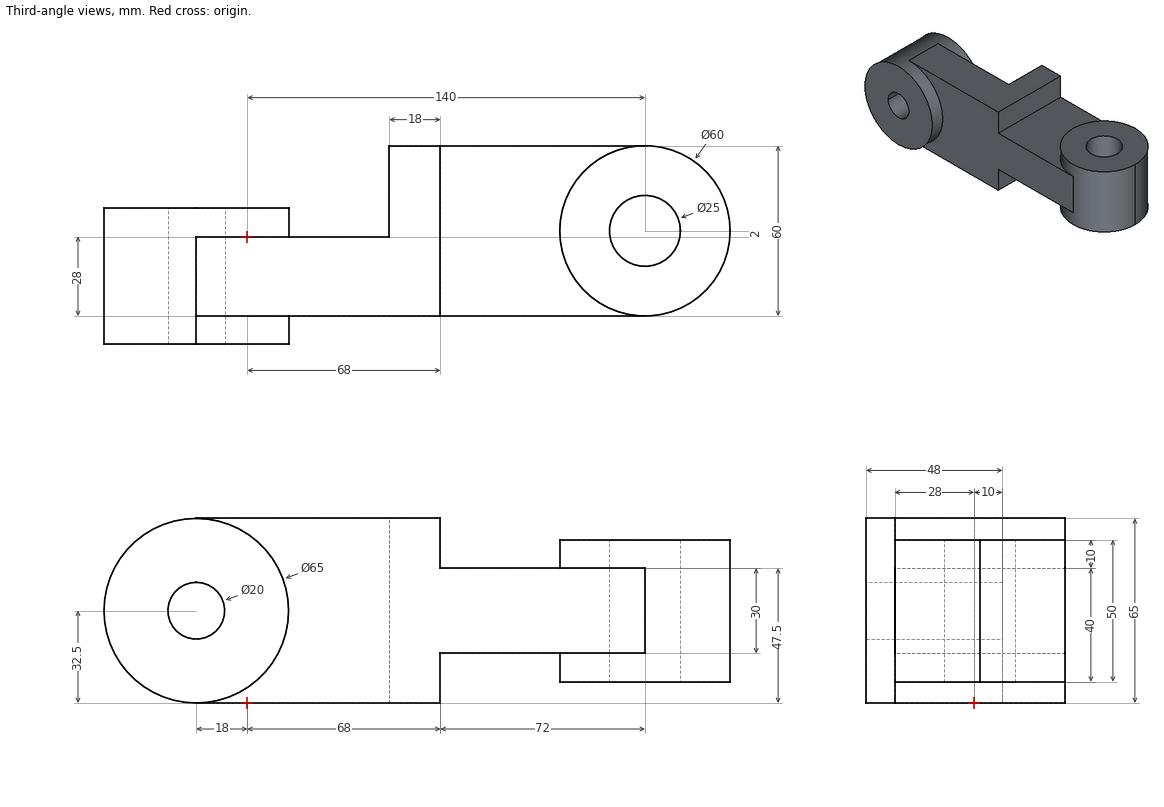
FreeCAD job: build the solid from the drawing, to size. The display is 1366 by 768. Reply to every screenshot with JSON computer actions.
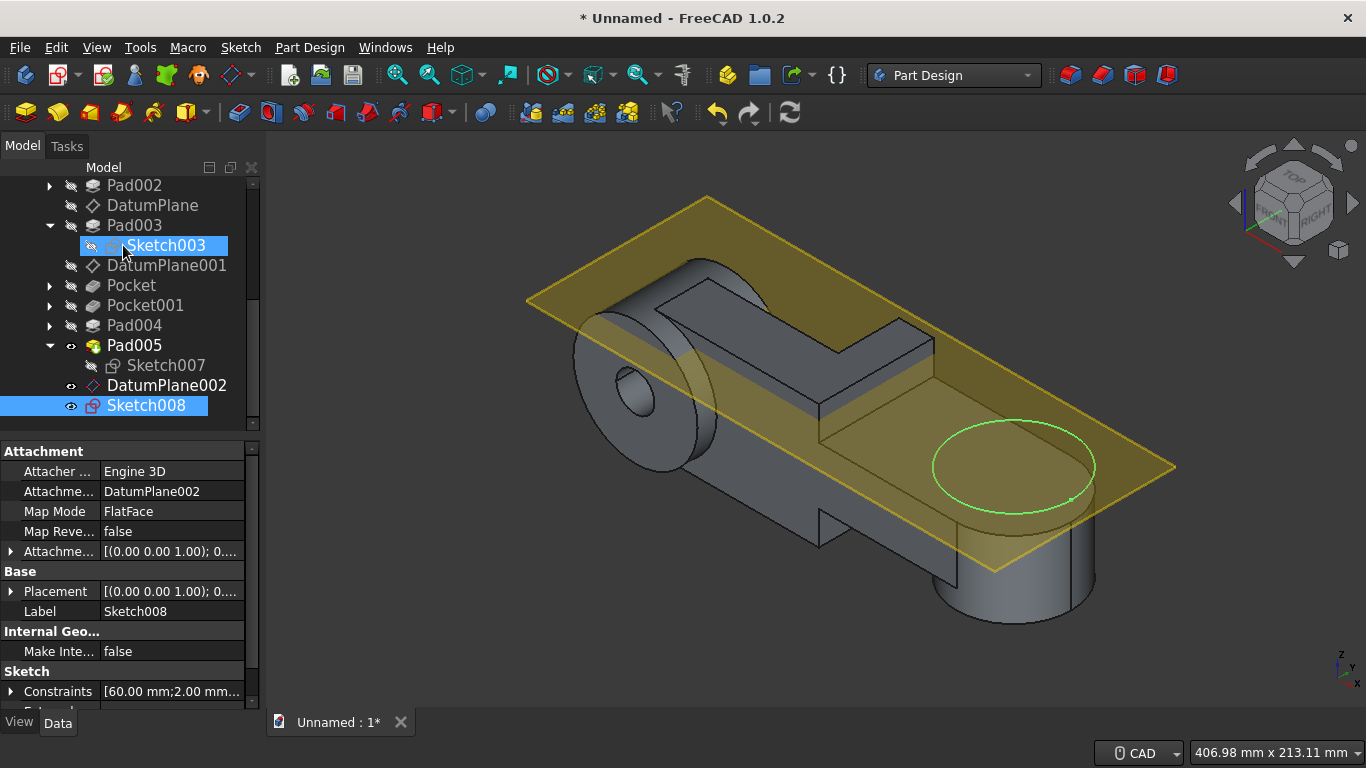
{"action": "left_click", "coordinate": [26, 112]}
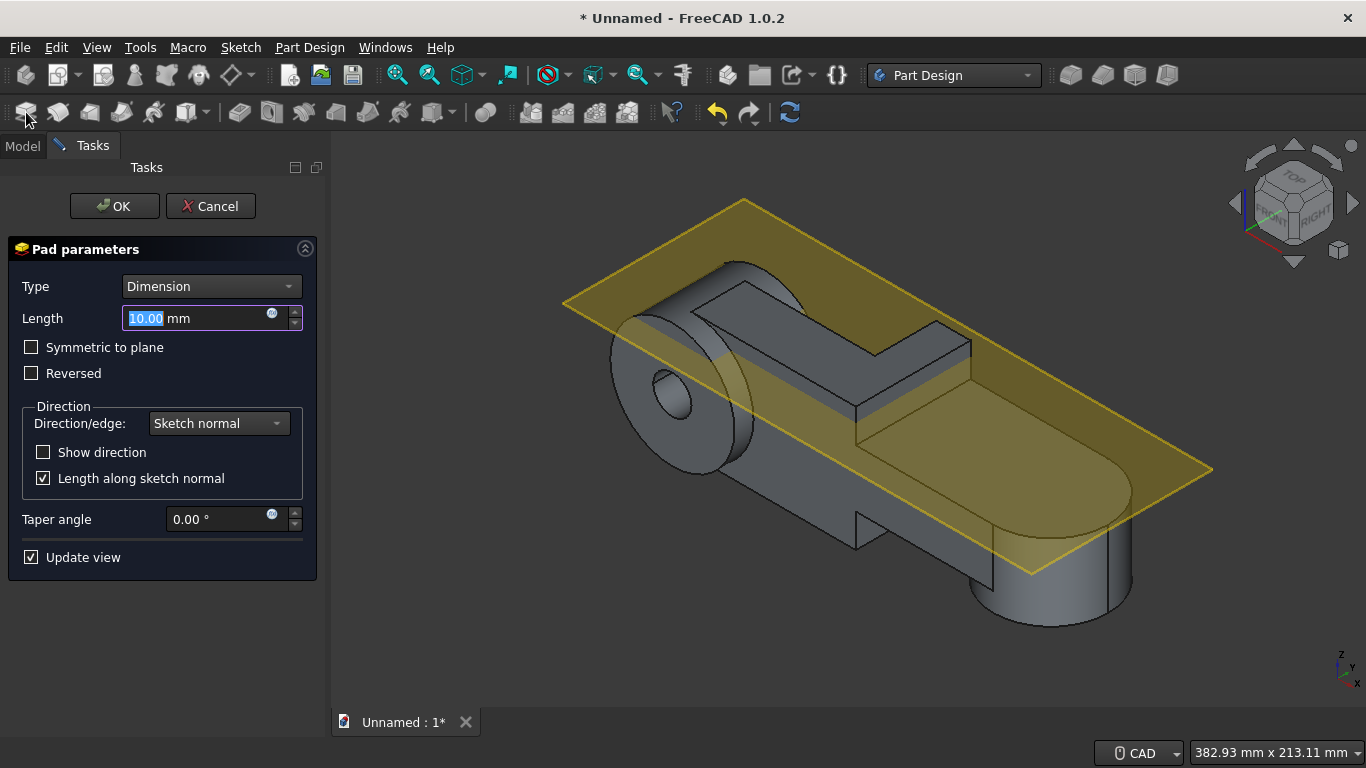
{"action": "type", "text": "10"}
{"action": "key", "text": "Tab"}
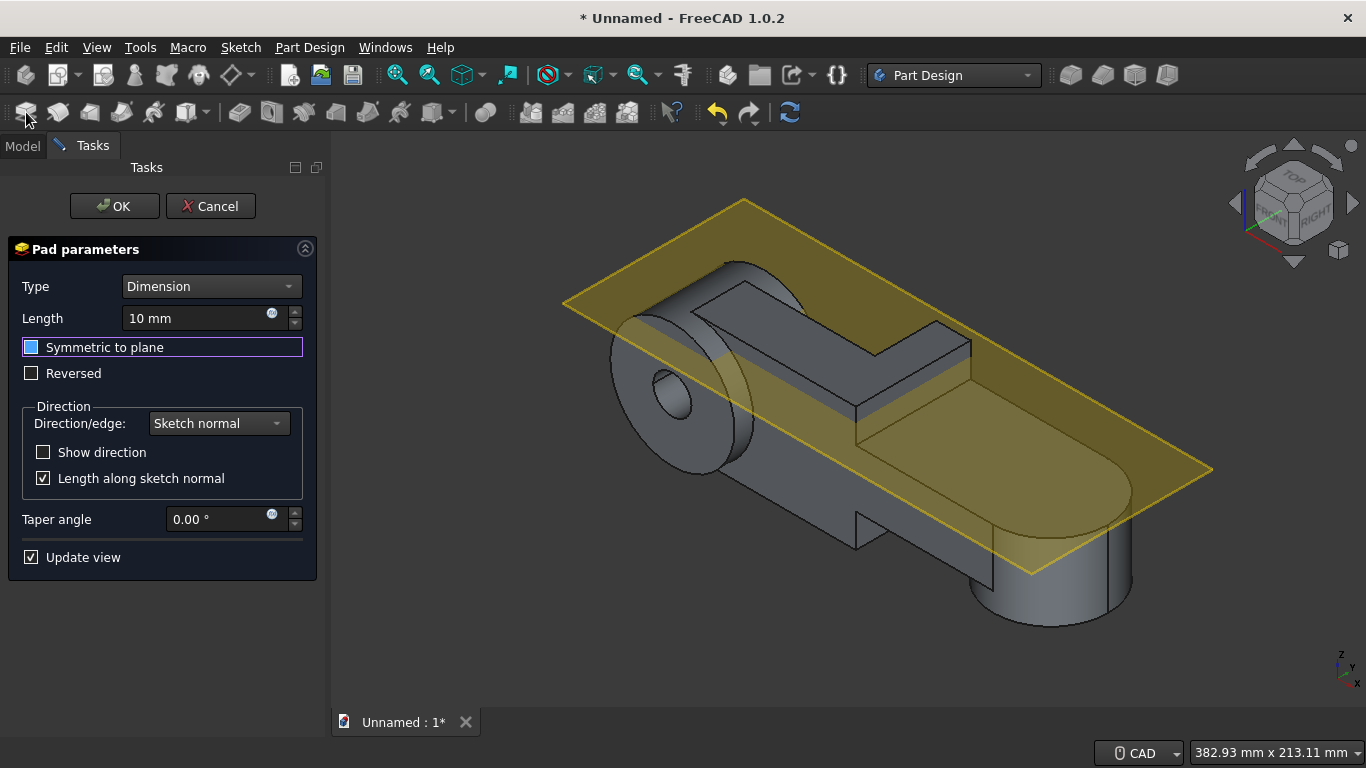
{"action": "left_click", "coordinate": [30, 373]}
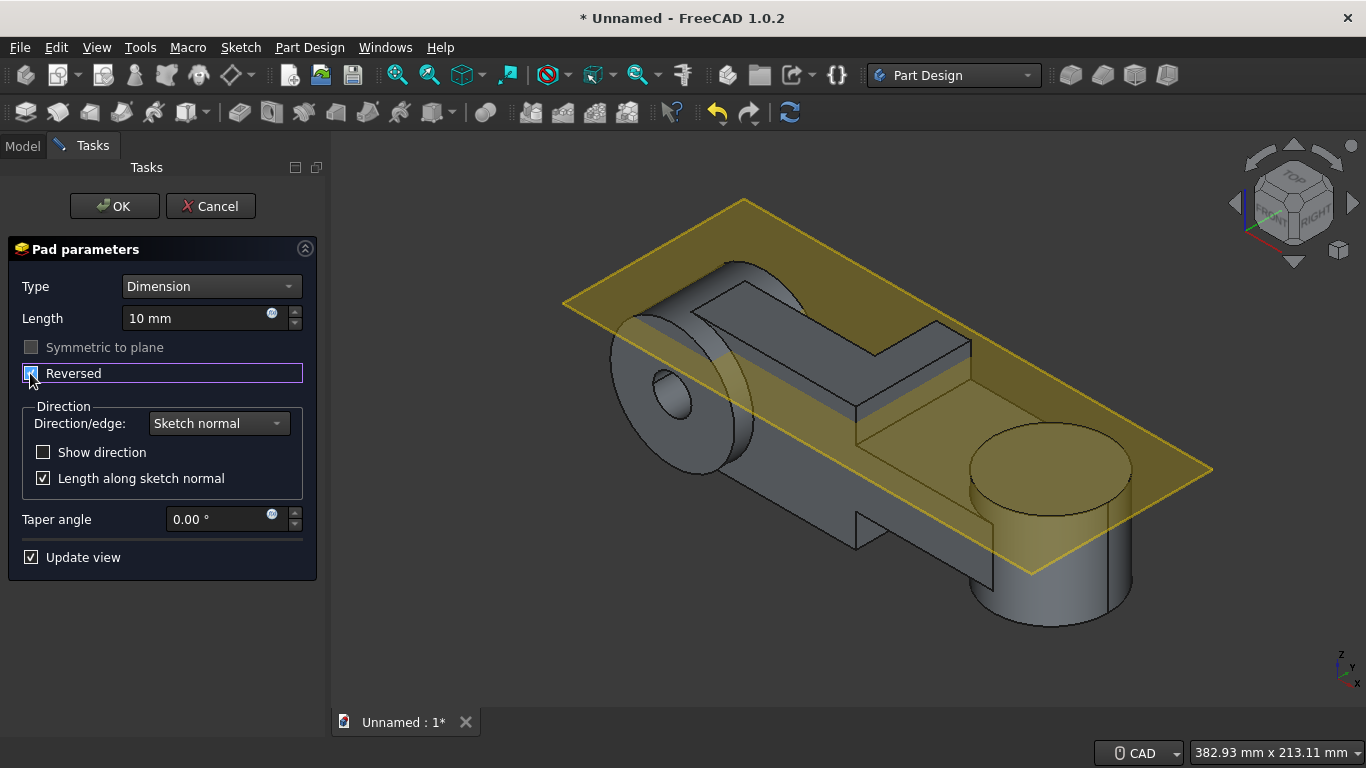
{"action": "left_click", "coordinate": [115, 206]}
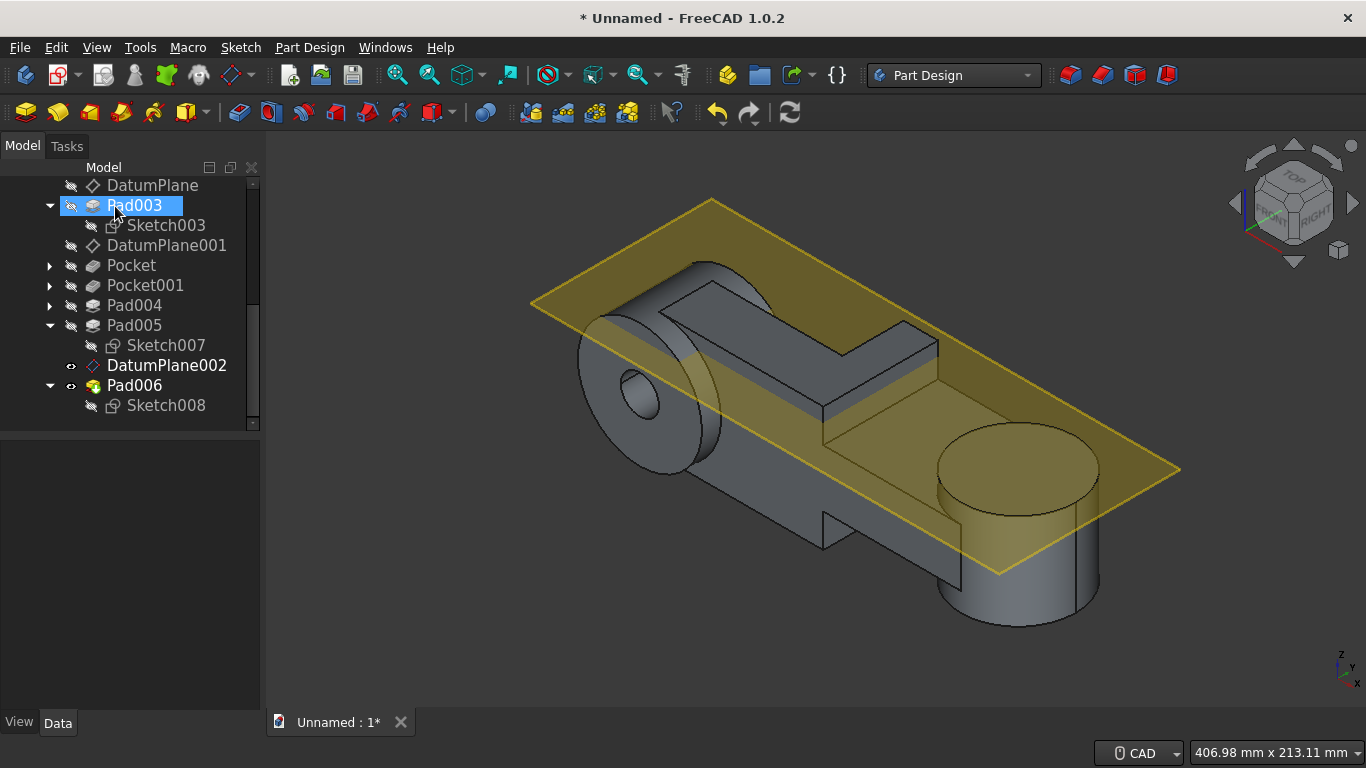
{"action": "left_click", "coordinate": [116, 366]}
{"action": "key", "text": "space"}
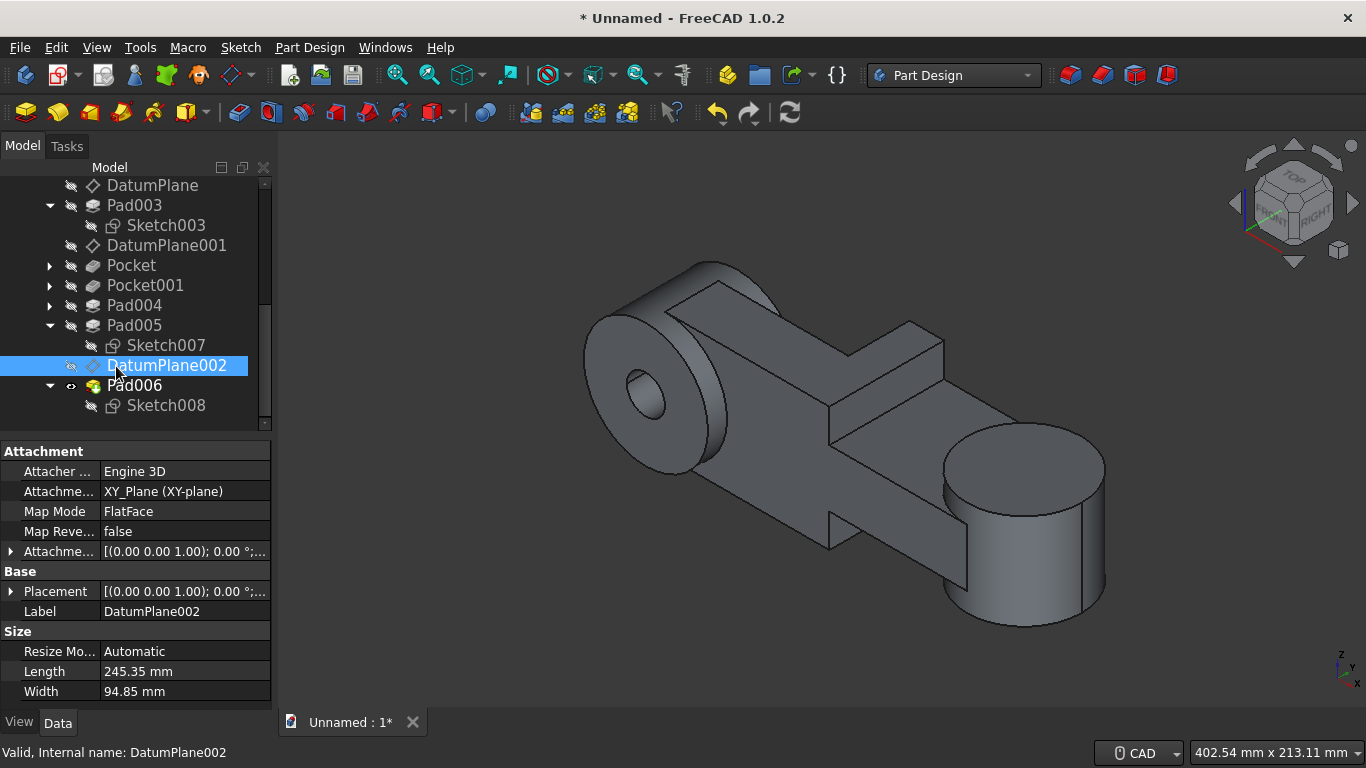
{"action": "left_click", "coordinate": [1024, 469]}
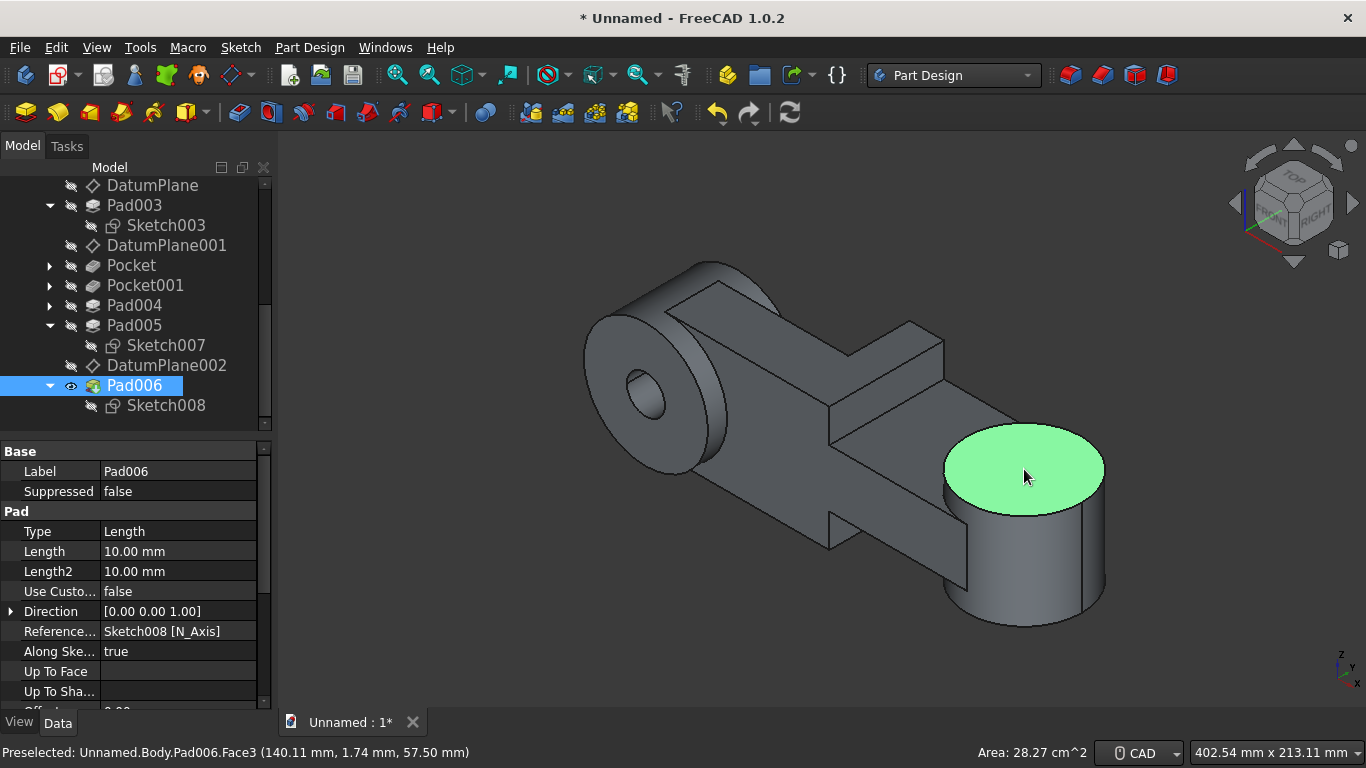
{"action": "left_click", "coordinate": [58, 76]}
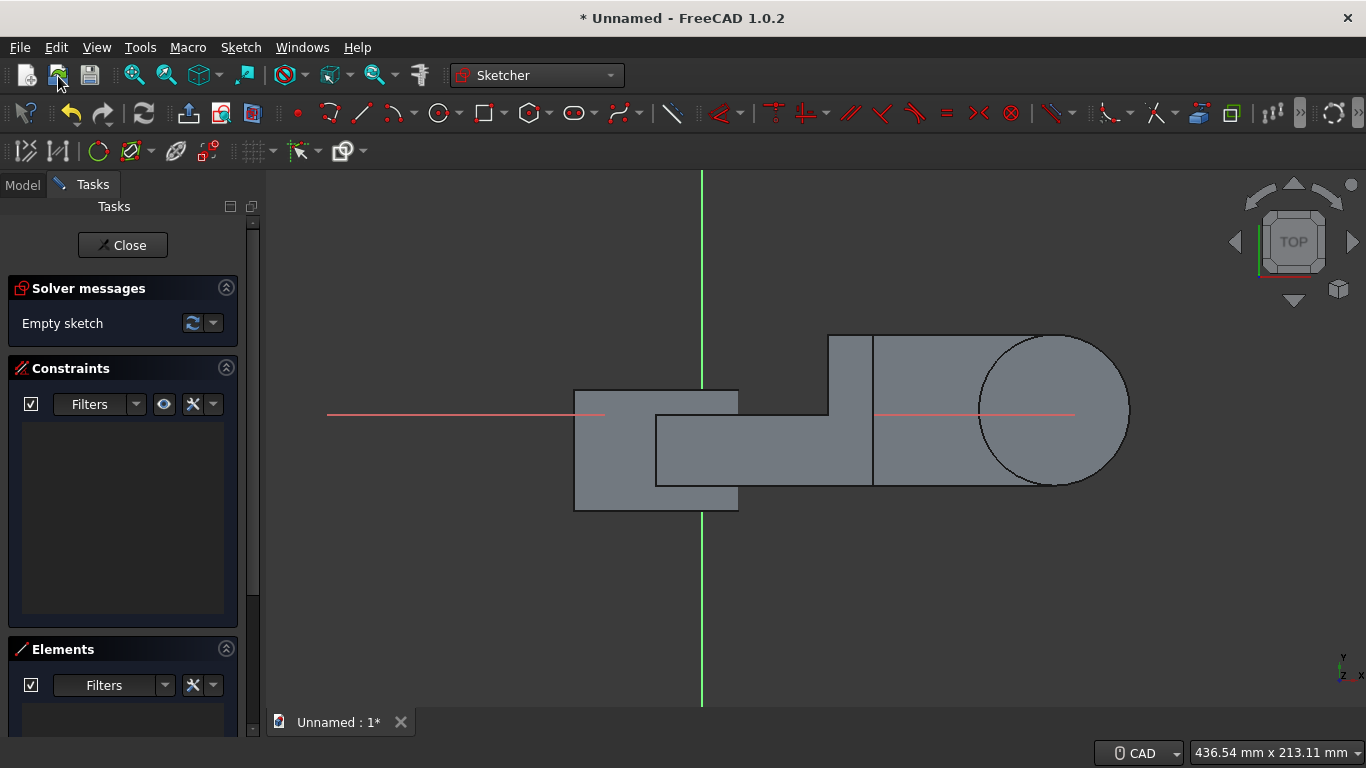
{"action": "scroll", "coordinate": [1132, 403], "scroll_direction": "up", "scroll_amount": 8}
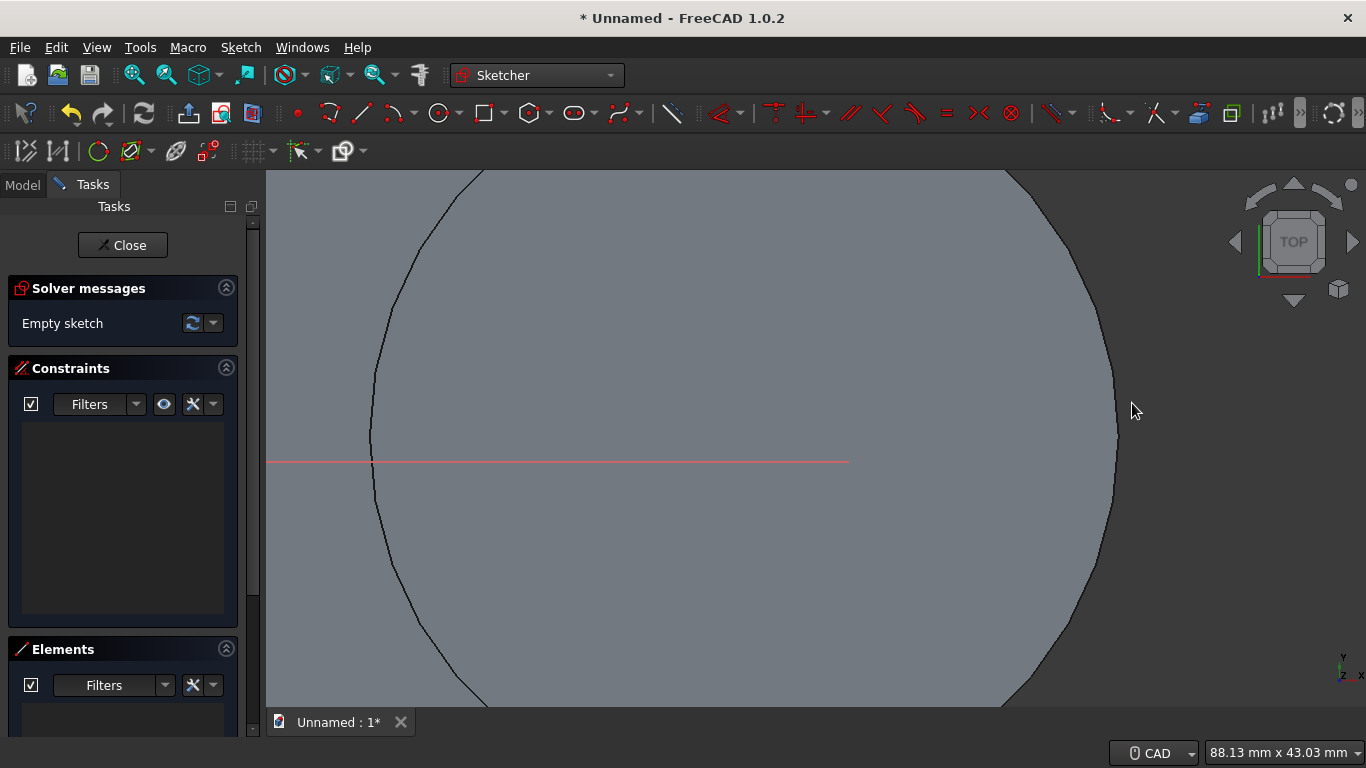
{"action": "key", "text": "g c"}